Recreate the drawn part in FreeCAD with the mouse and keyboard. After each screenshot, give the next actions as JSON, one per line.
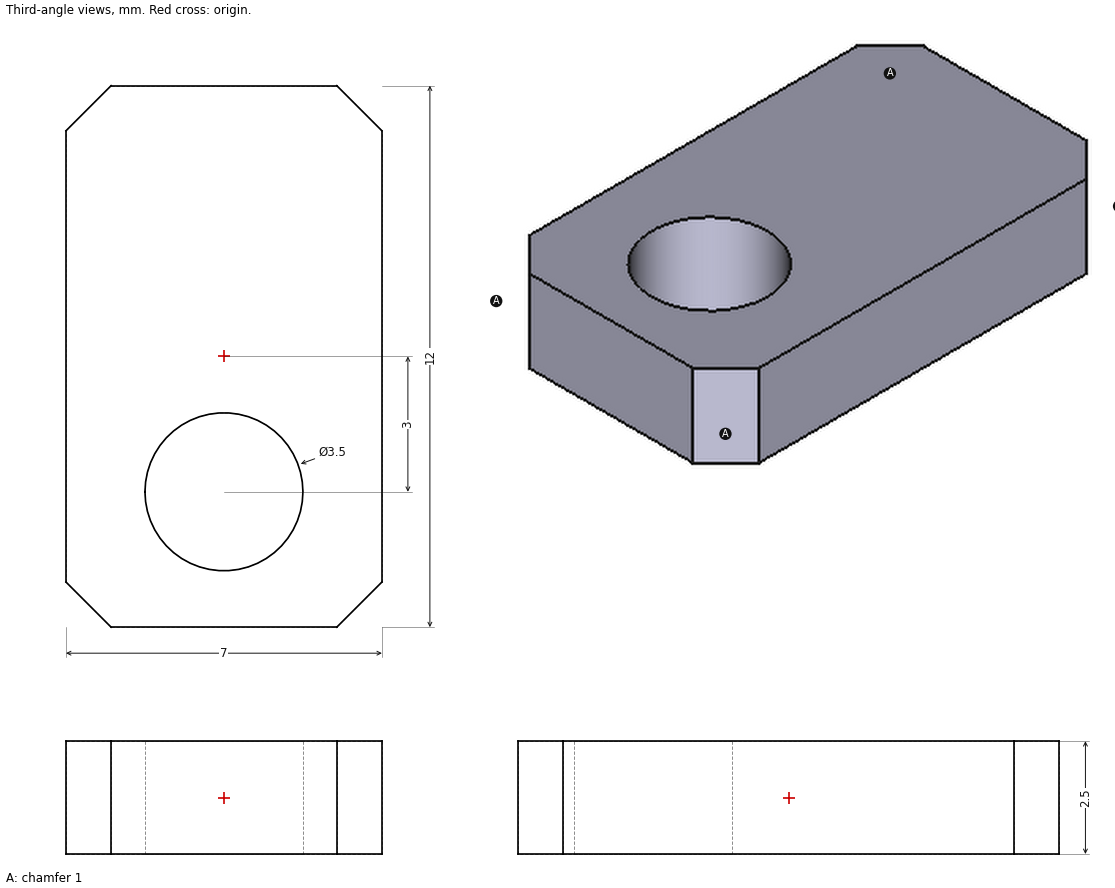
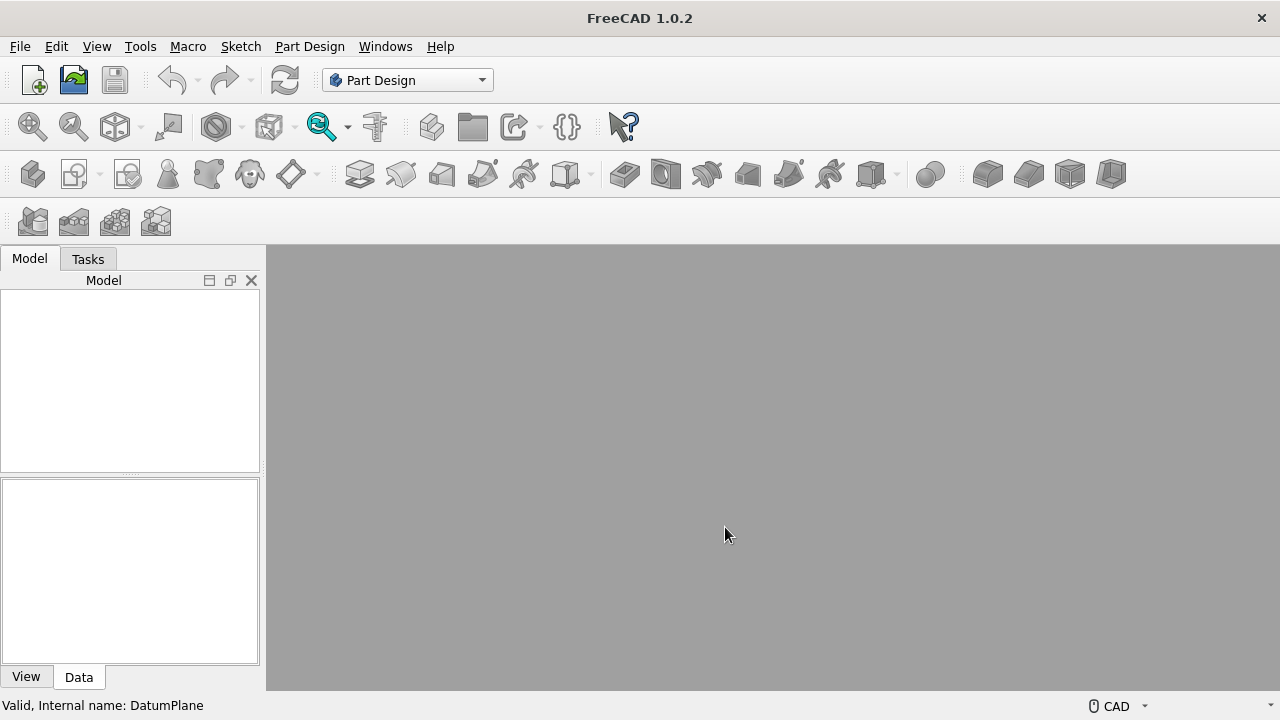
{"action": "left_click", "coordinate": [33, 80]}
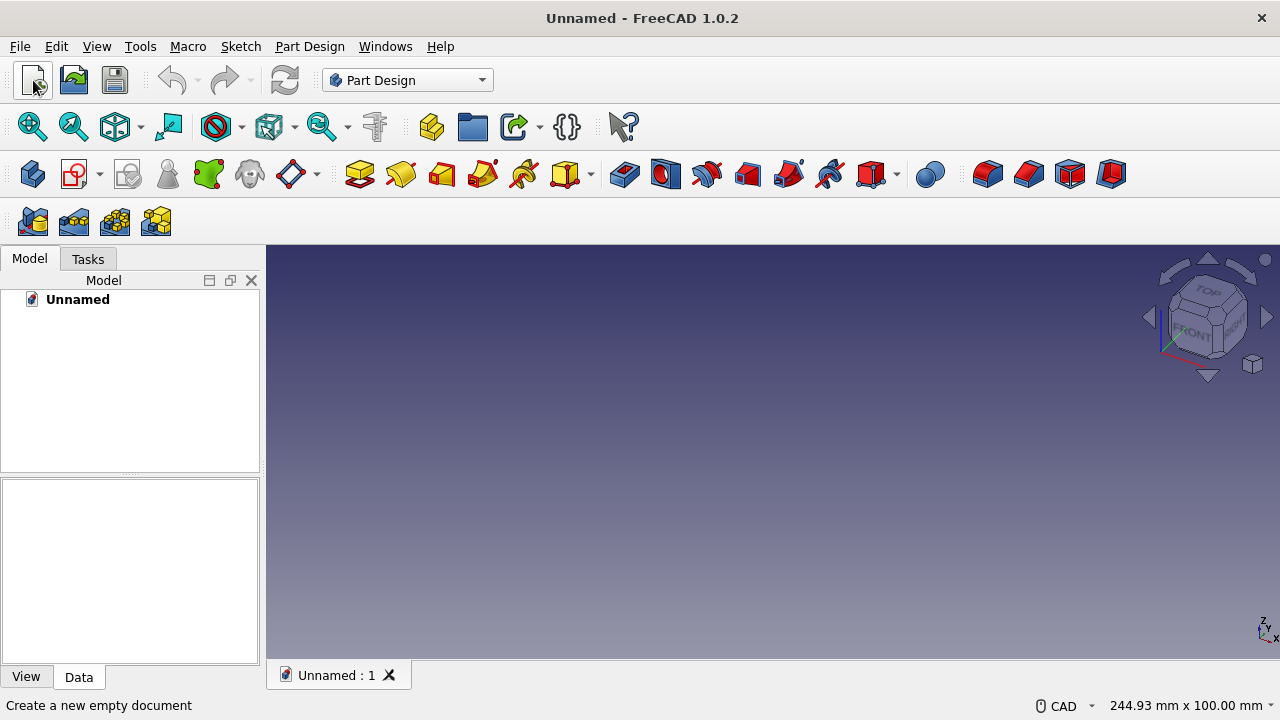
{"action": "left_click", "coordinate": [74, 174]}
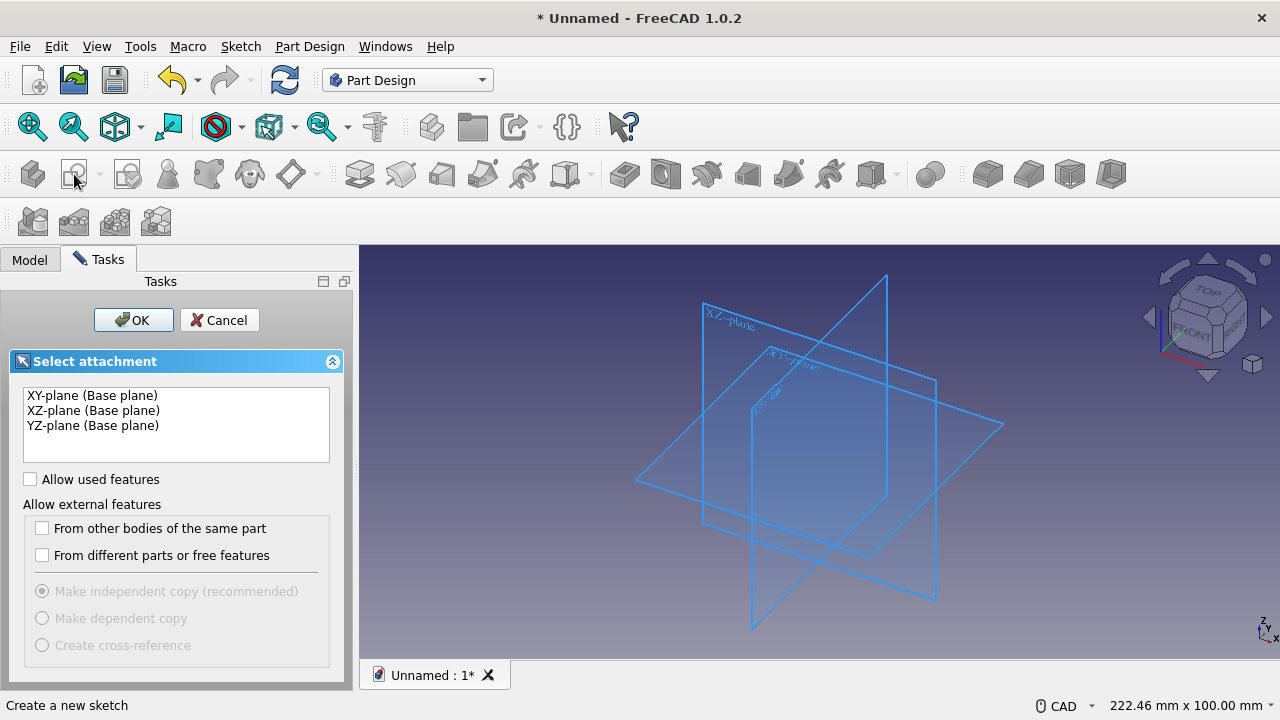
{"action": "left_click", "coordinate": [84, 396]}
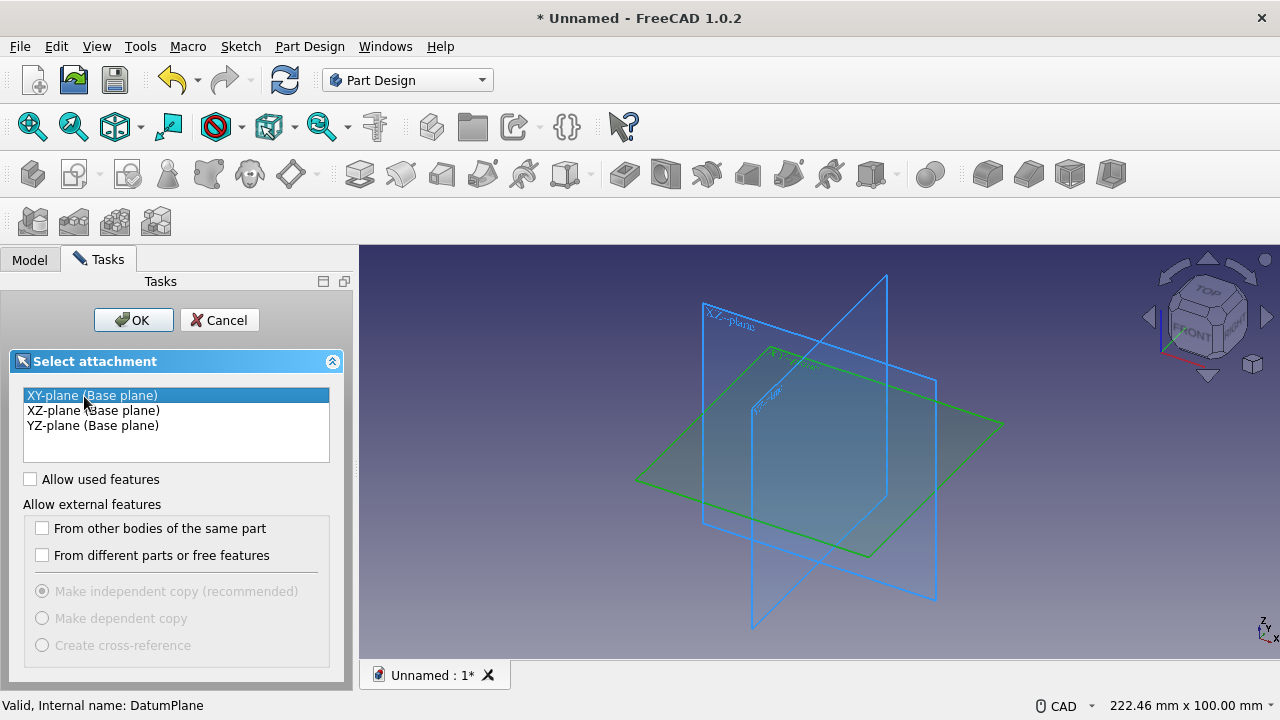
{"action": "left_click", "coordinate": [134, 320]}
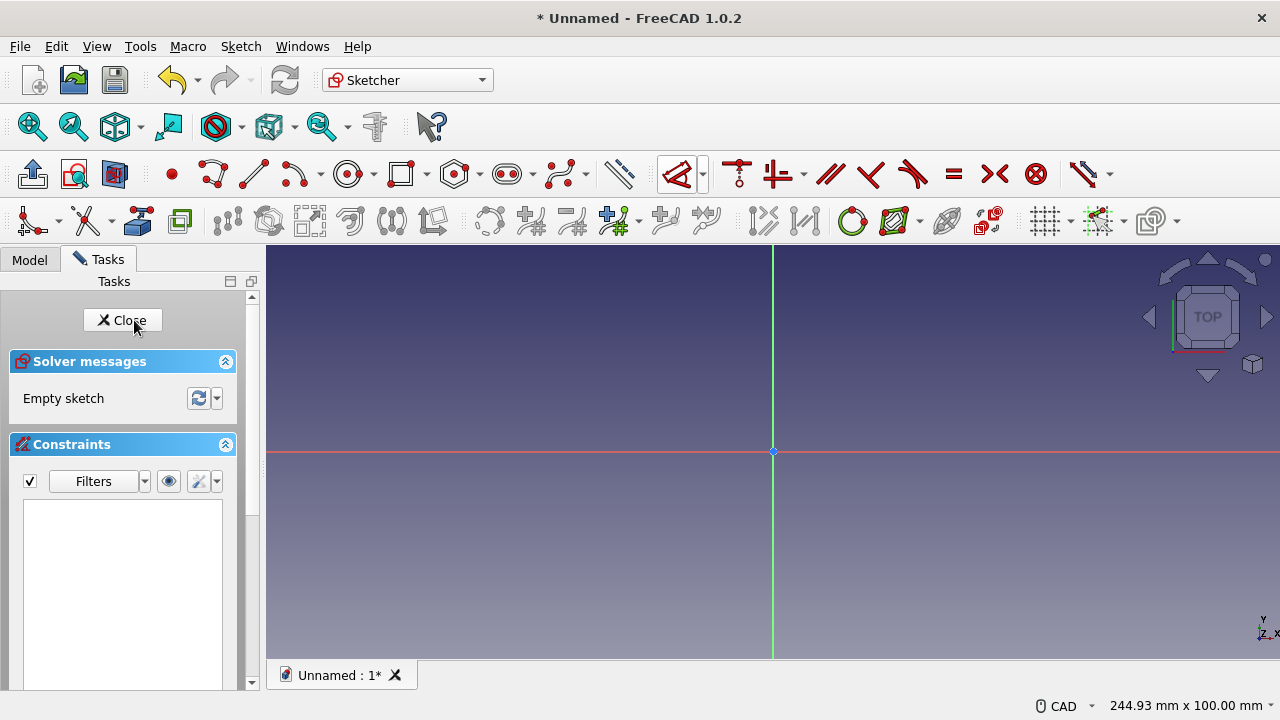
{"action": "scroll", "coordinate": [790, 452], "scroll_direction": "up", "scroll_amount": 8}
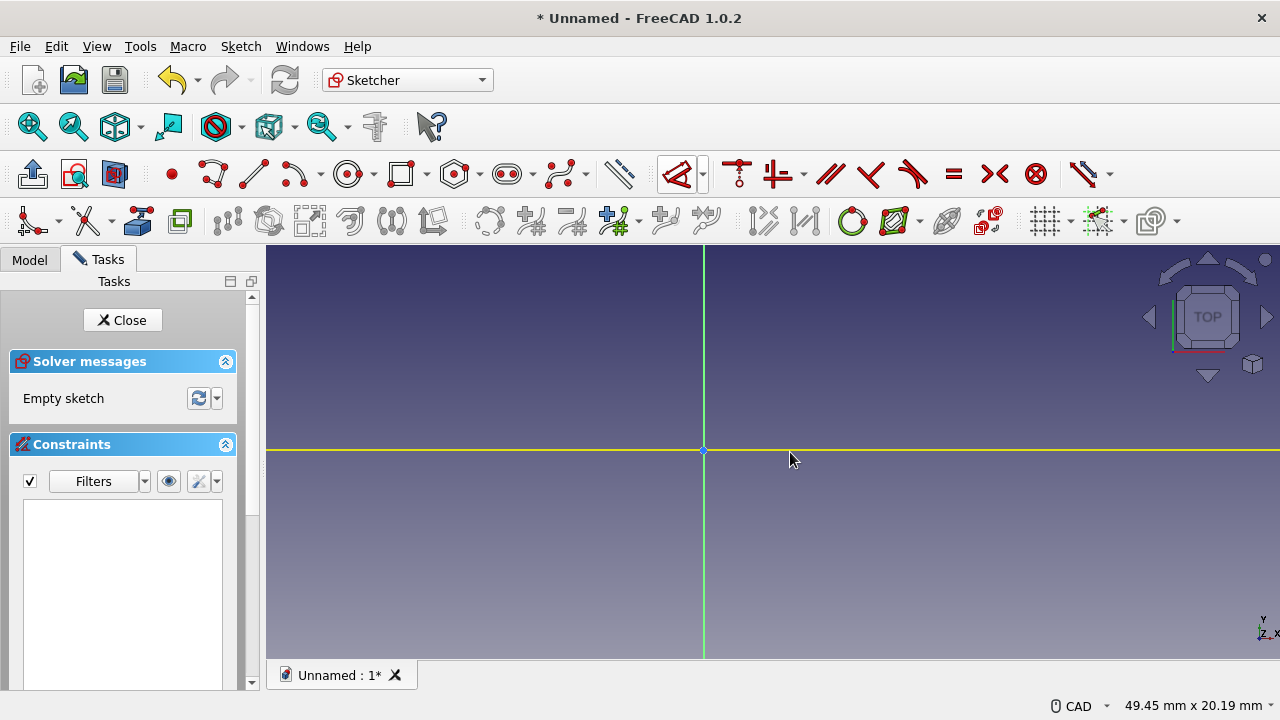
{"action": "key", "text": "g v"}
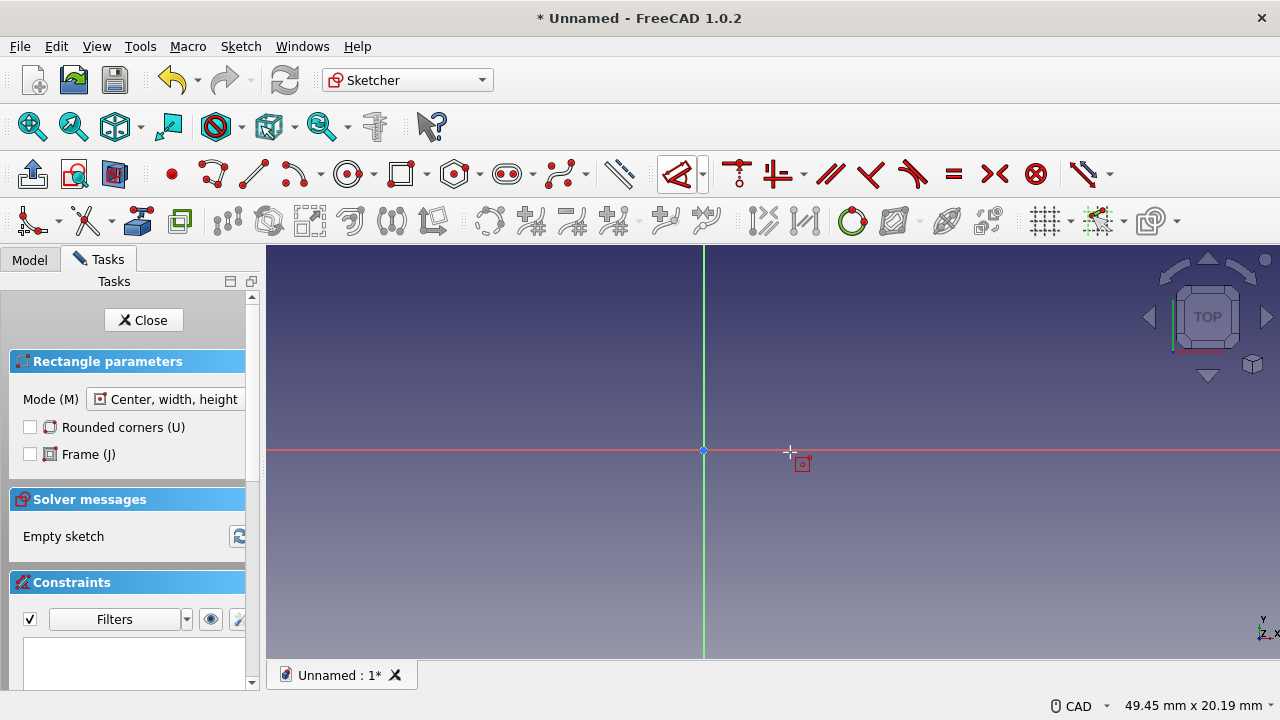
{"action": "left_click", "coordinate": [704, 450]}
{"action": "left_click", "coordinate": [776, 327]}
{"action": "key", "text": "Escape"}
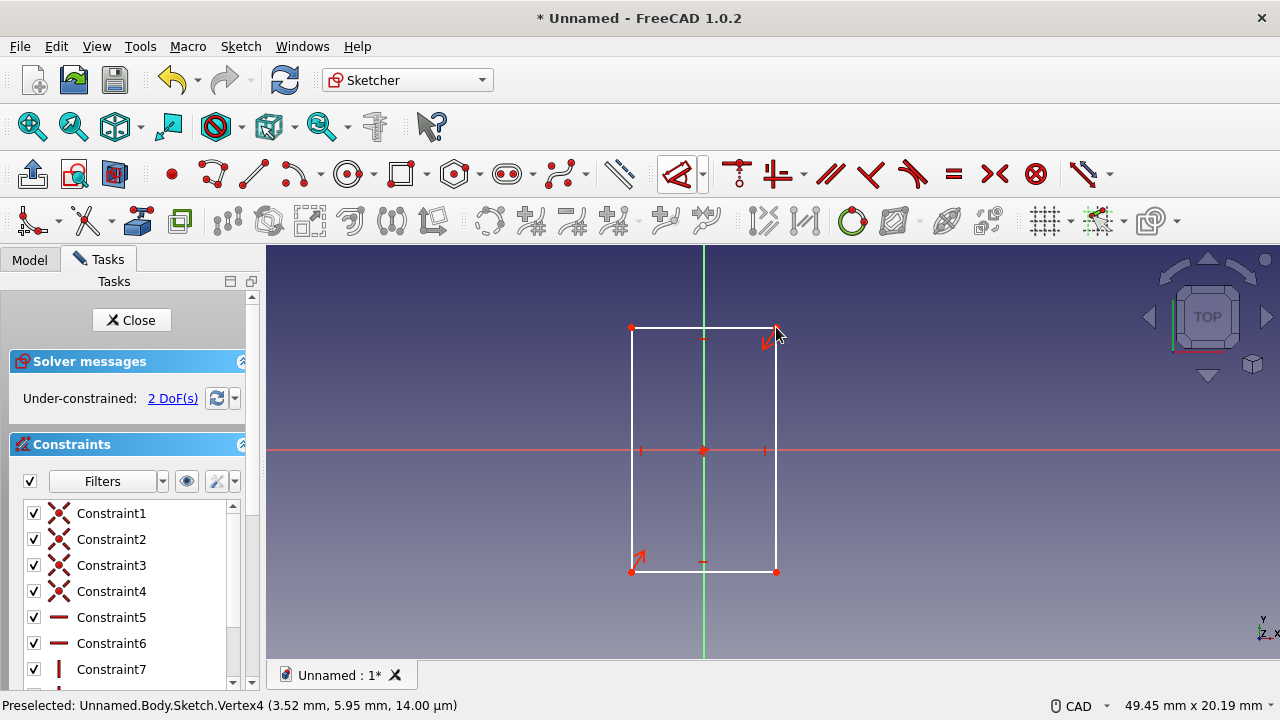
{"action": "left_click", "coordinate": [676, 174]}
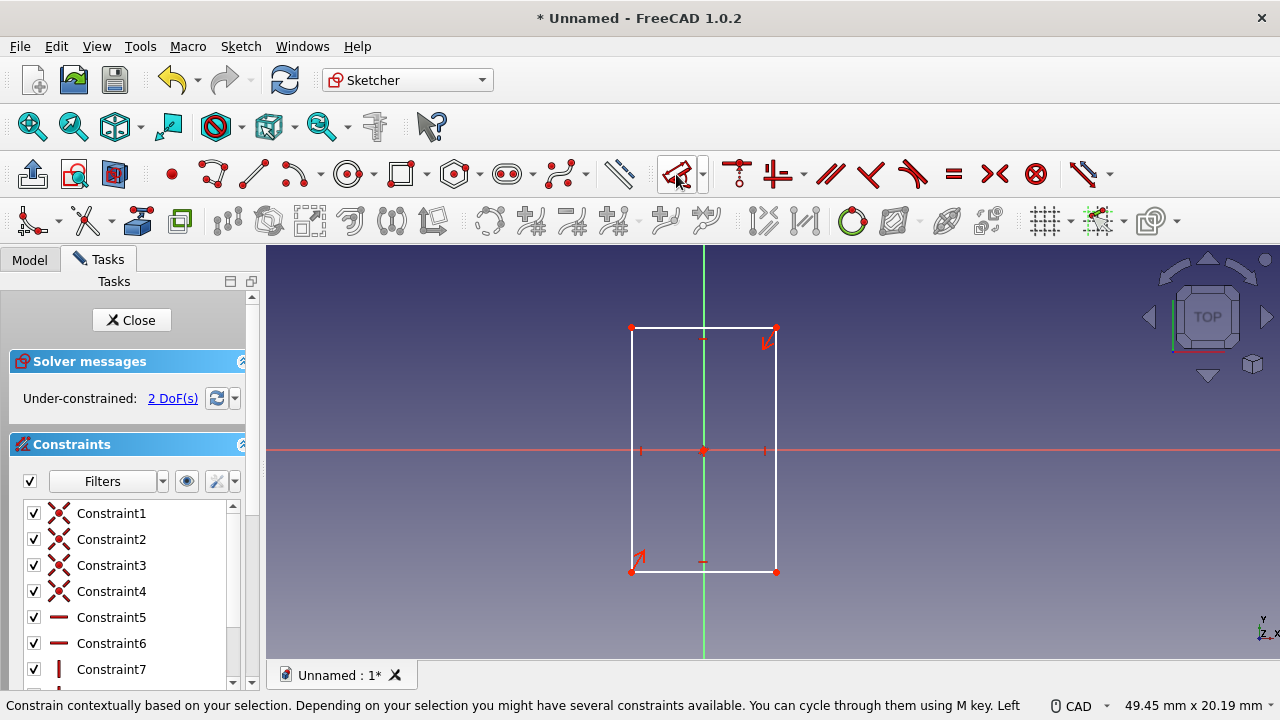
{"action": "left_click", "coordinate": [675, 572]}
{"action": "left_click", "coordinate": [671, 606]}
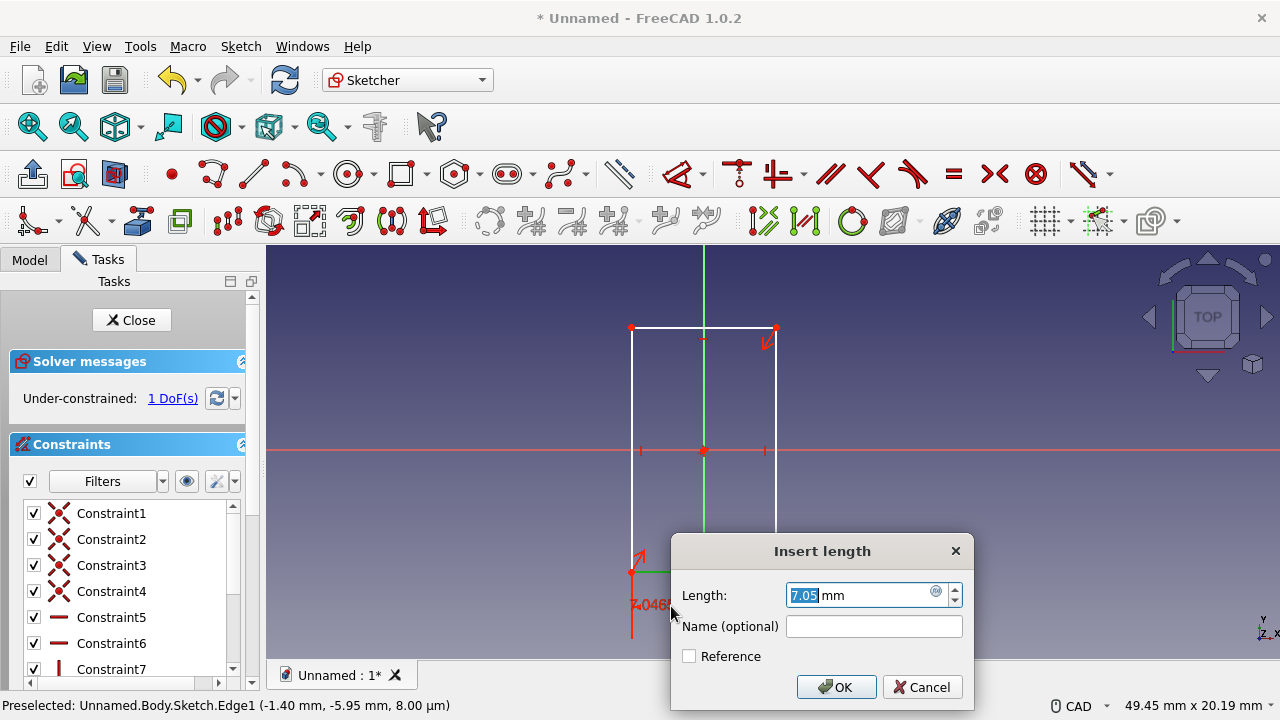
{"action": "type", "text": "7"}
{"action": "key", "text": "Return"}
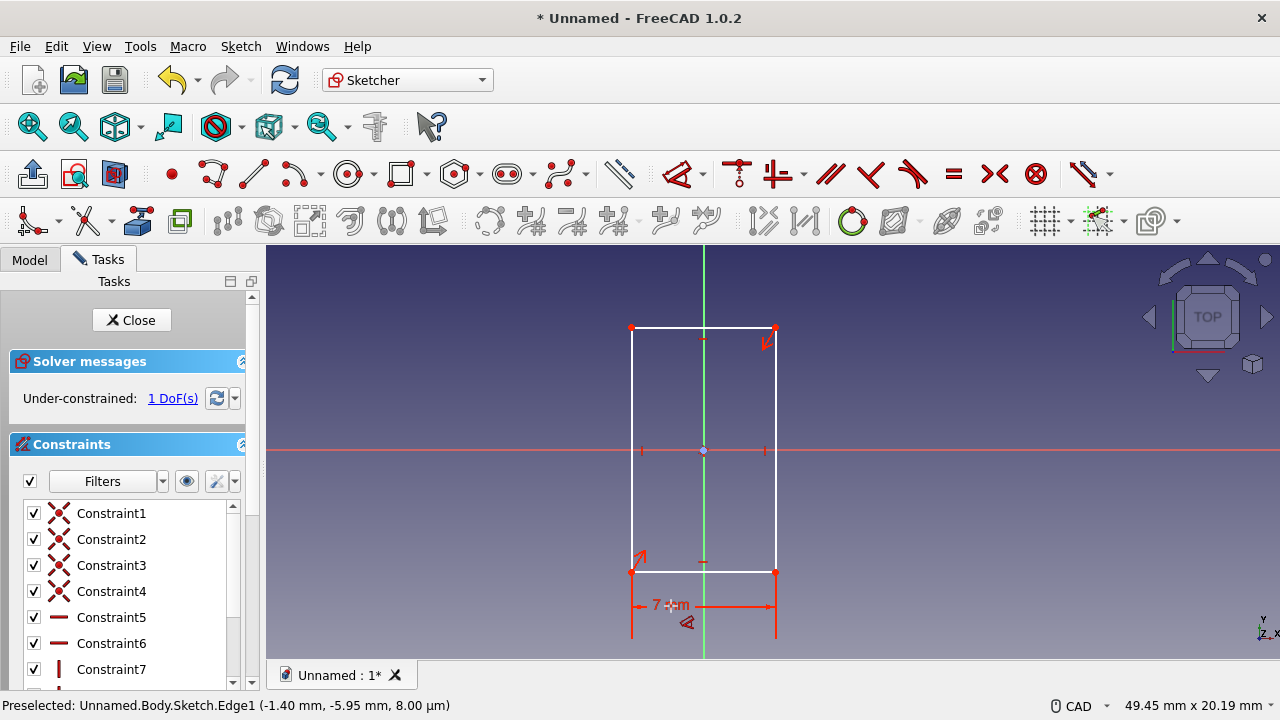
{"action": "left_click", "coordinate": [776, 499]}
{"action": "left_click", "coordinate": [810, 394]}